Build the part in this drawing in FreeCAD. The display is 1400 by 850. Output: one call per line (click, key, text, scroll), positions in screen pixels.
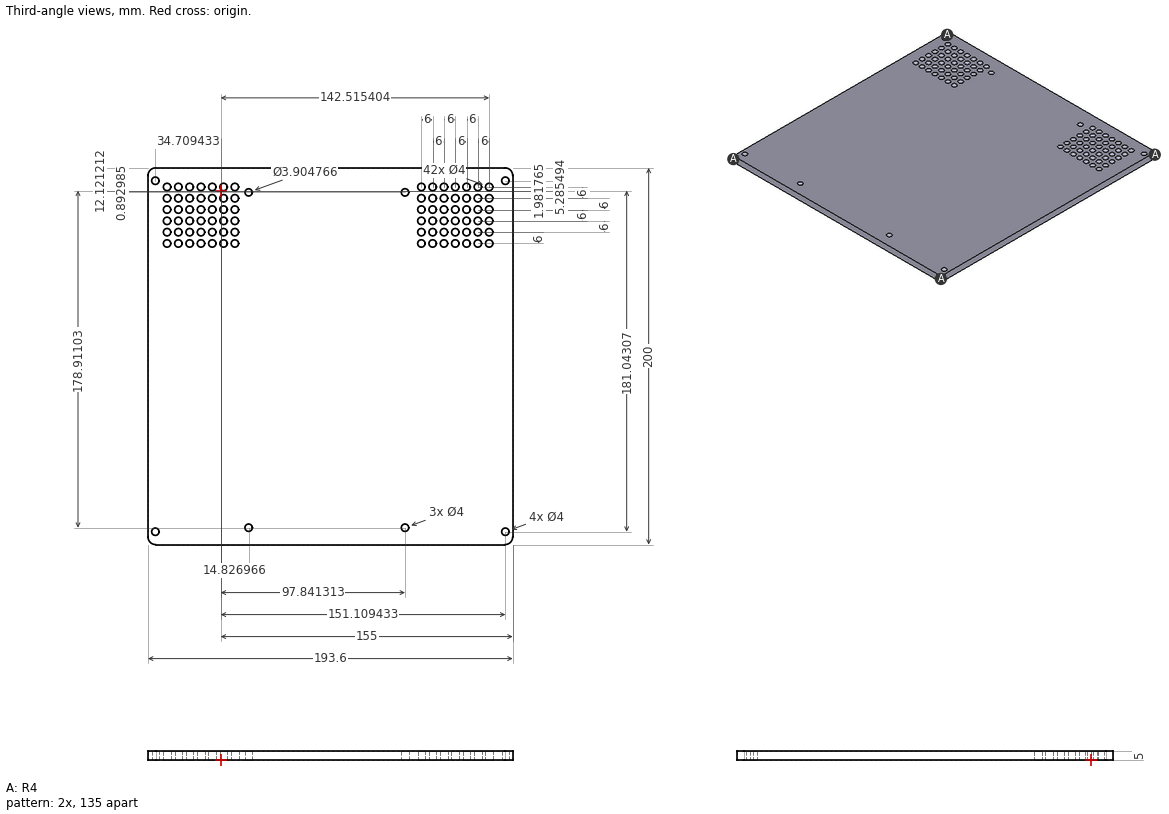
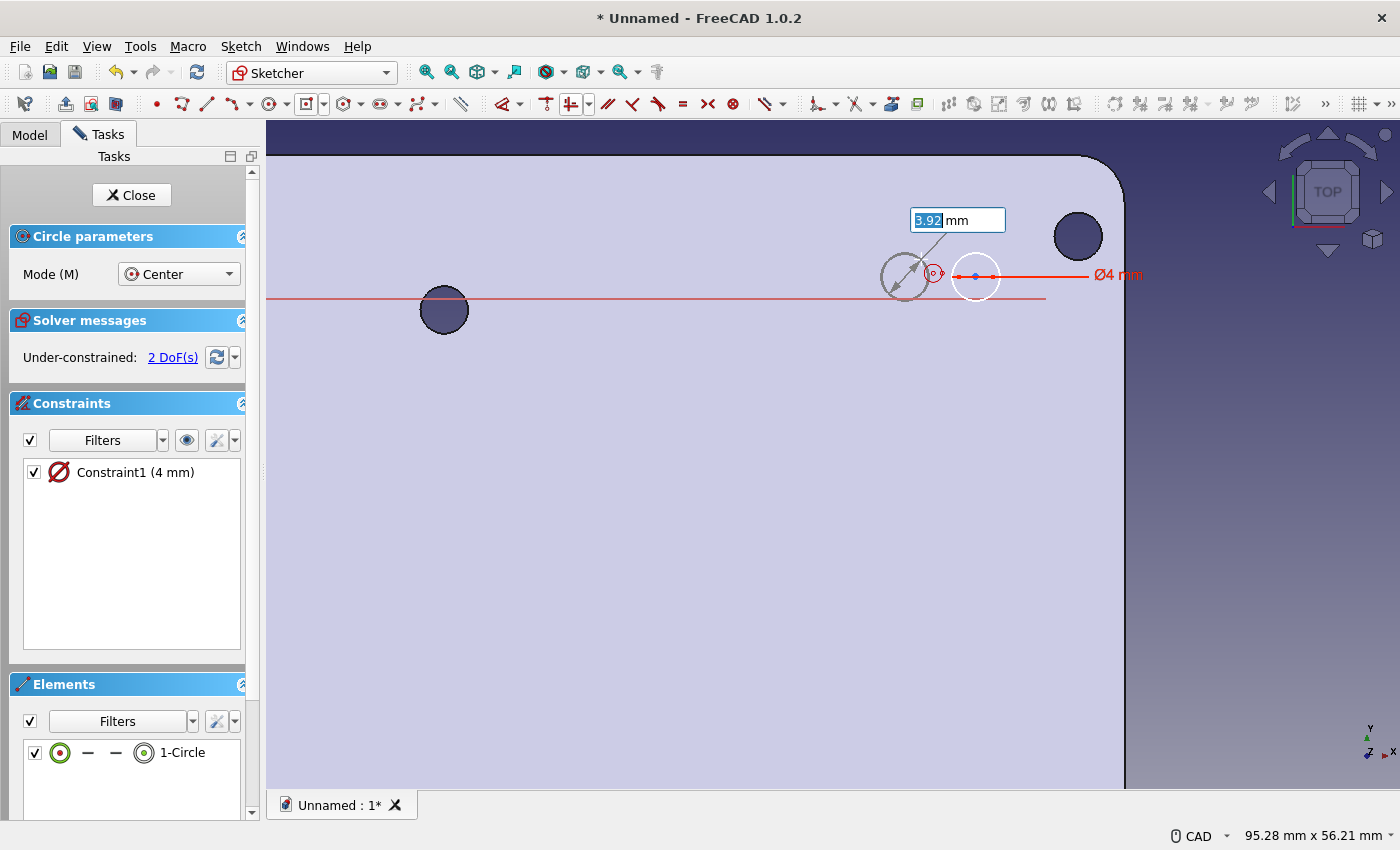
text(4)
key(Return)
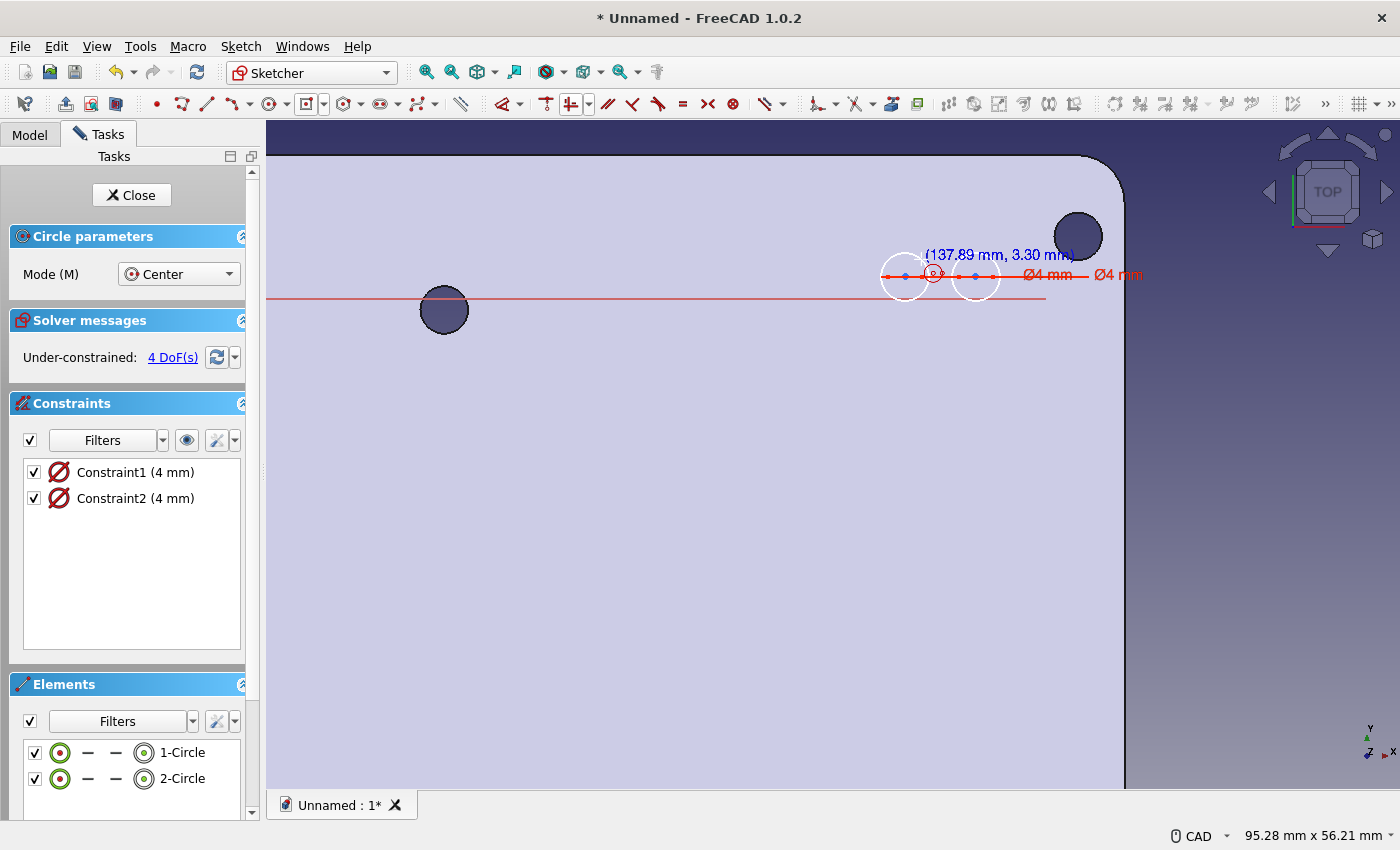
click(833, 276)
move(850, 259)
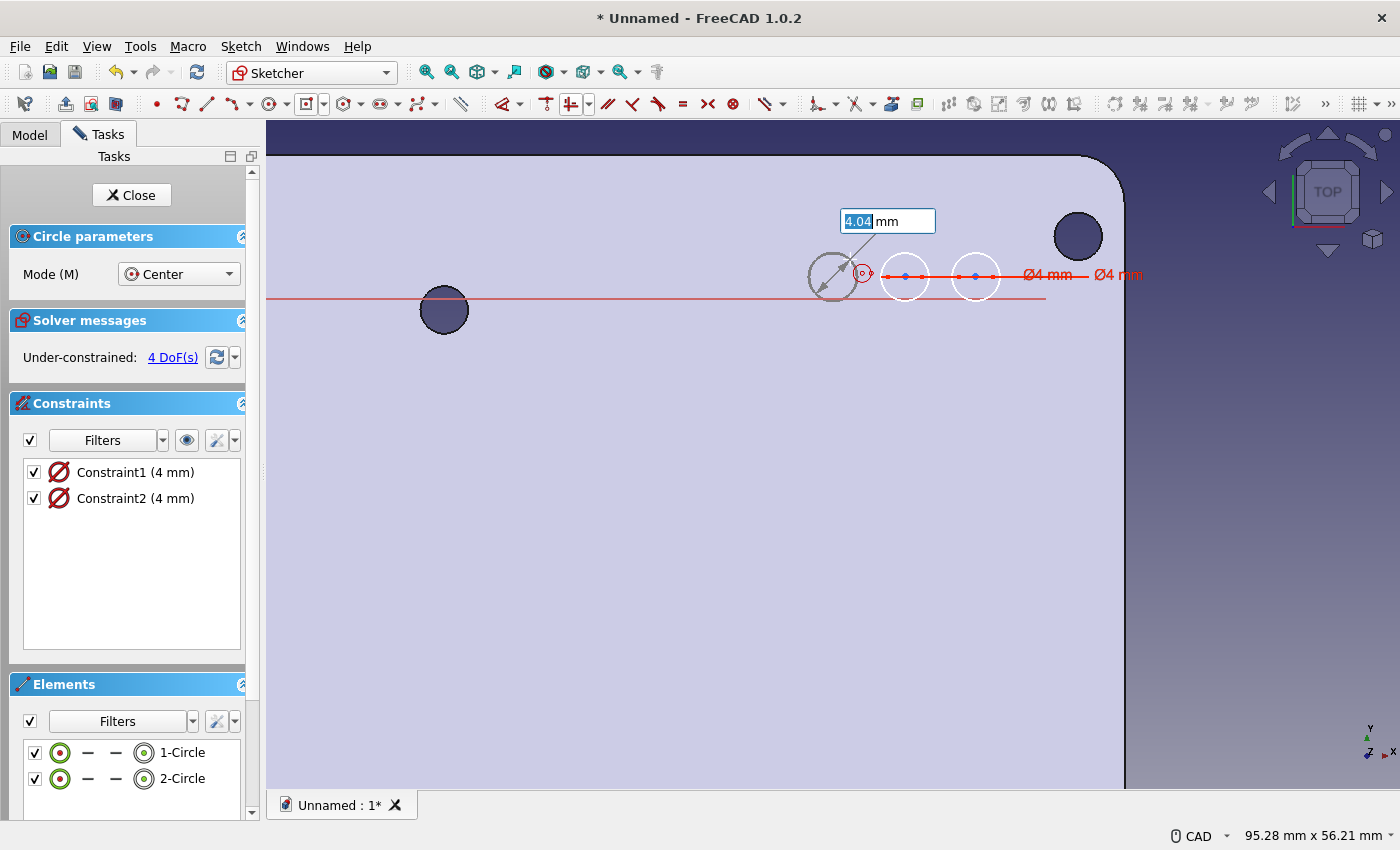
text(4)
key(Return)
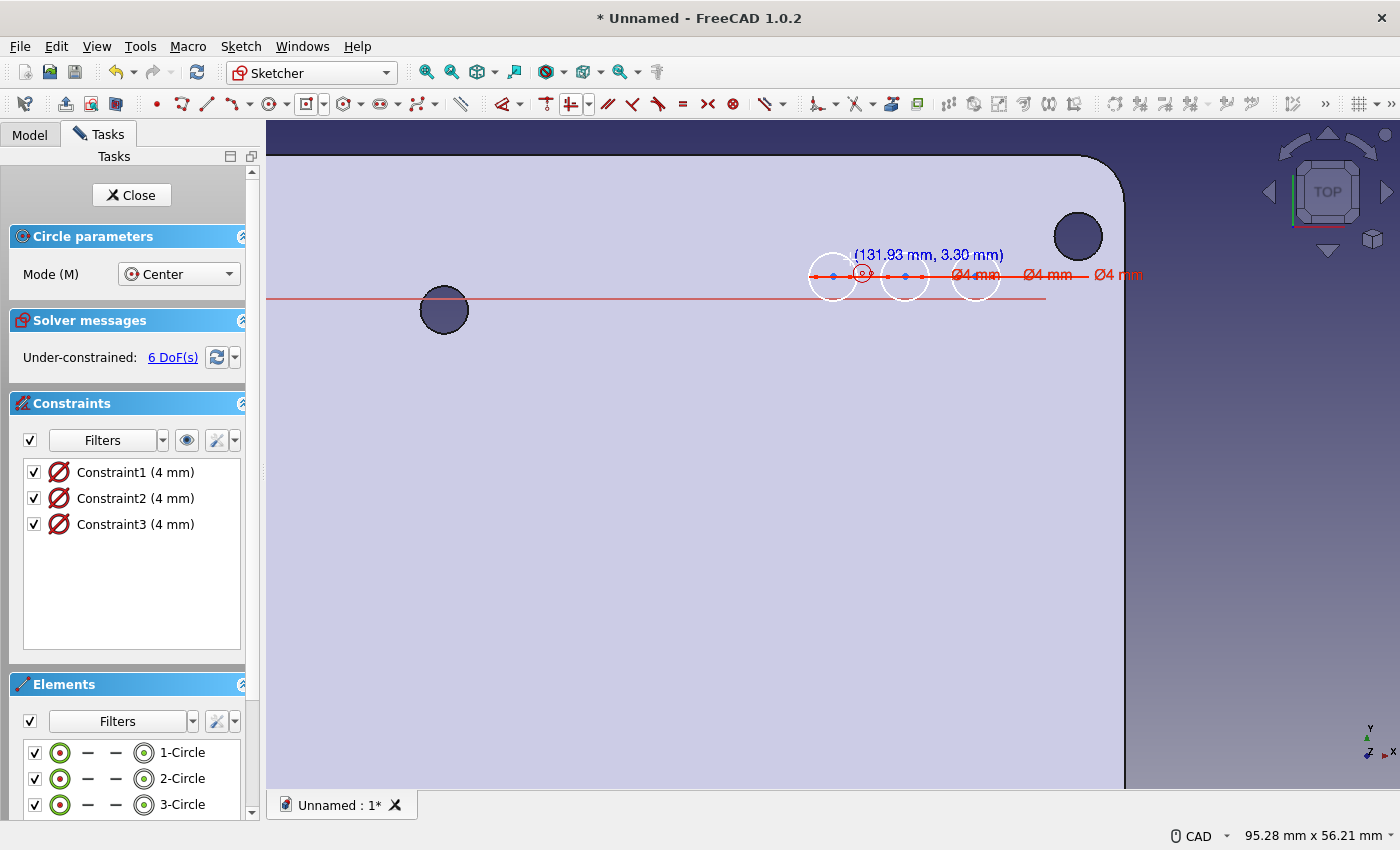
click(762, 276)
move(779, 259)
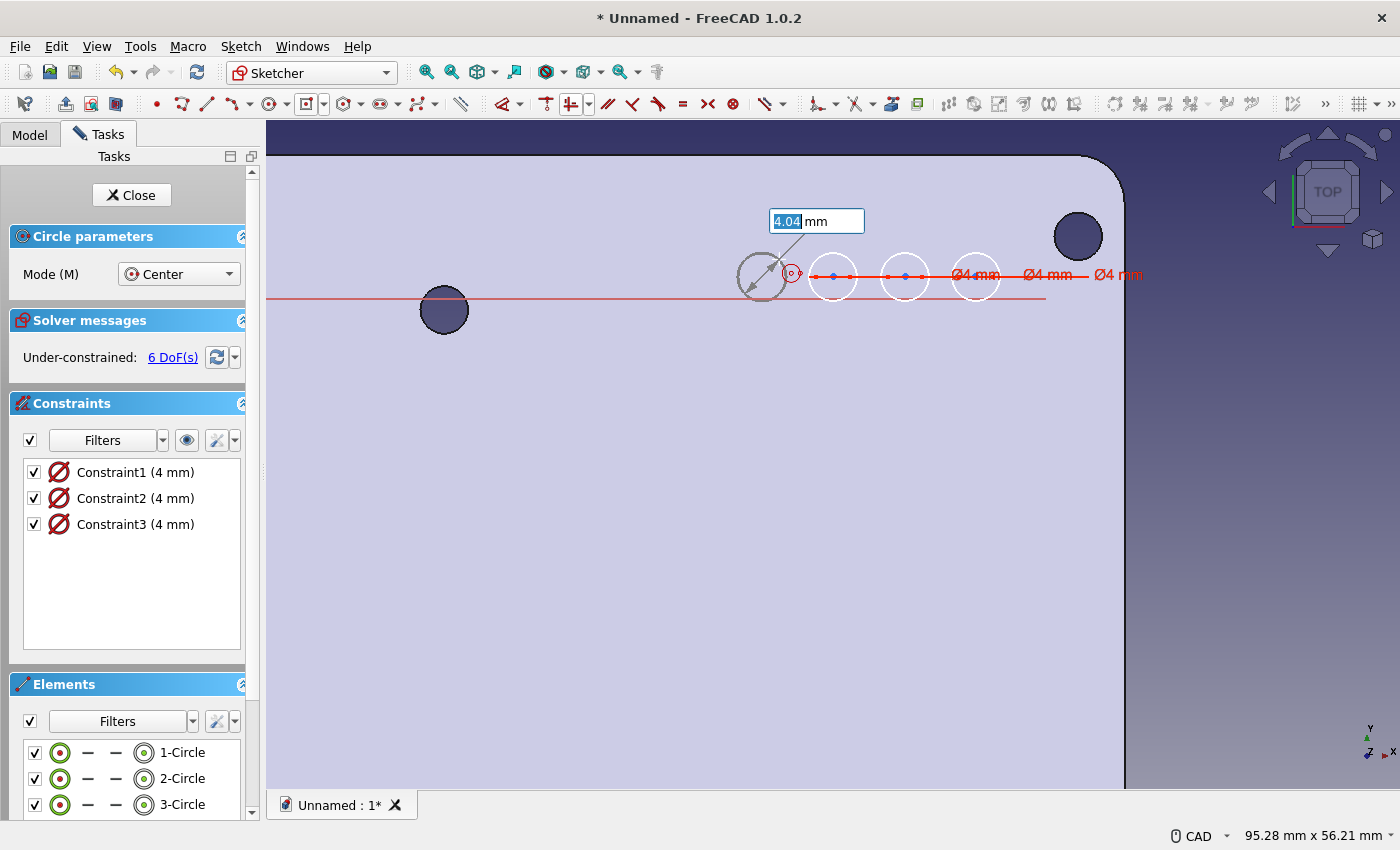
text(4)
key(Return)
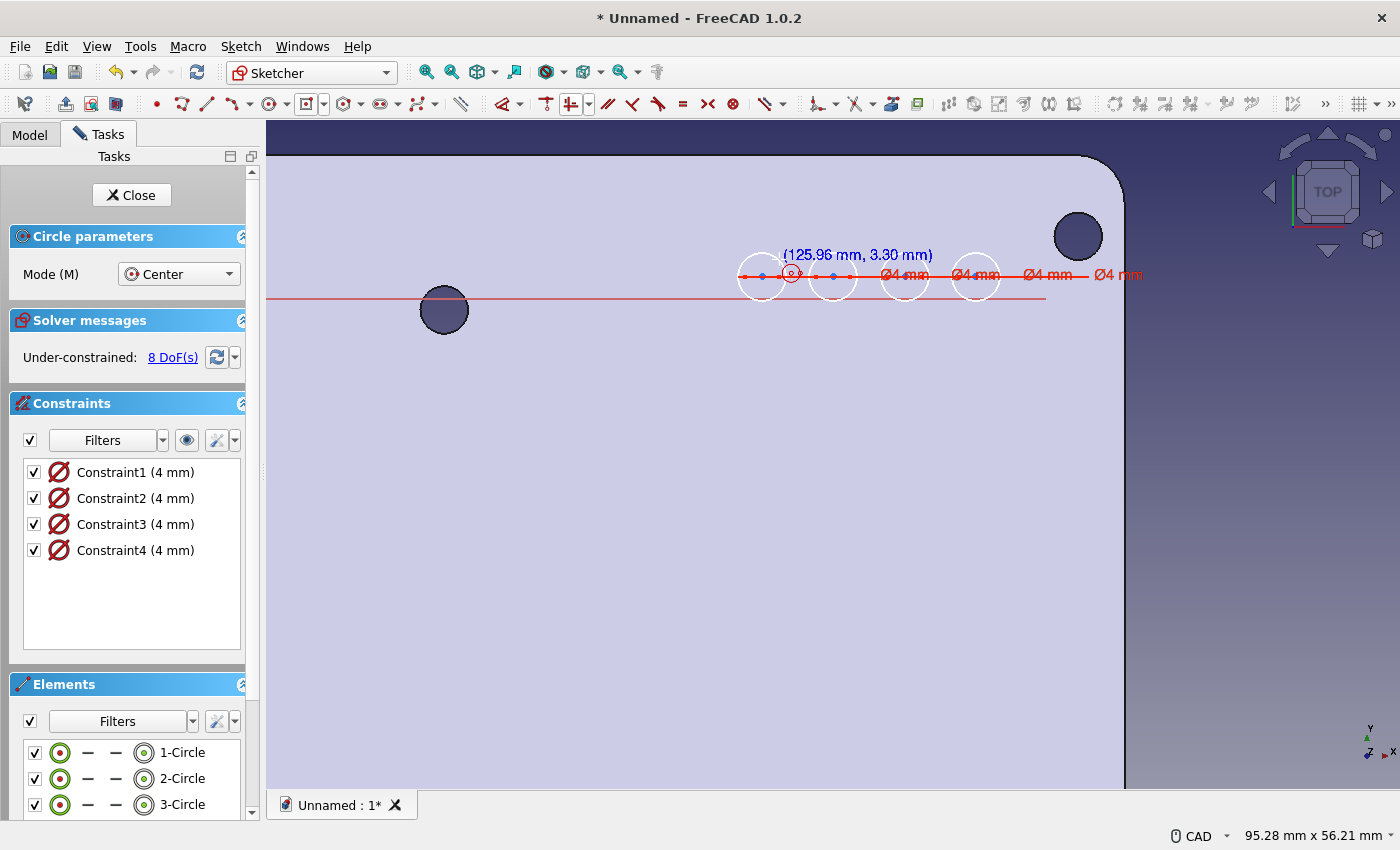
click(690, 276)
move(707, 259)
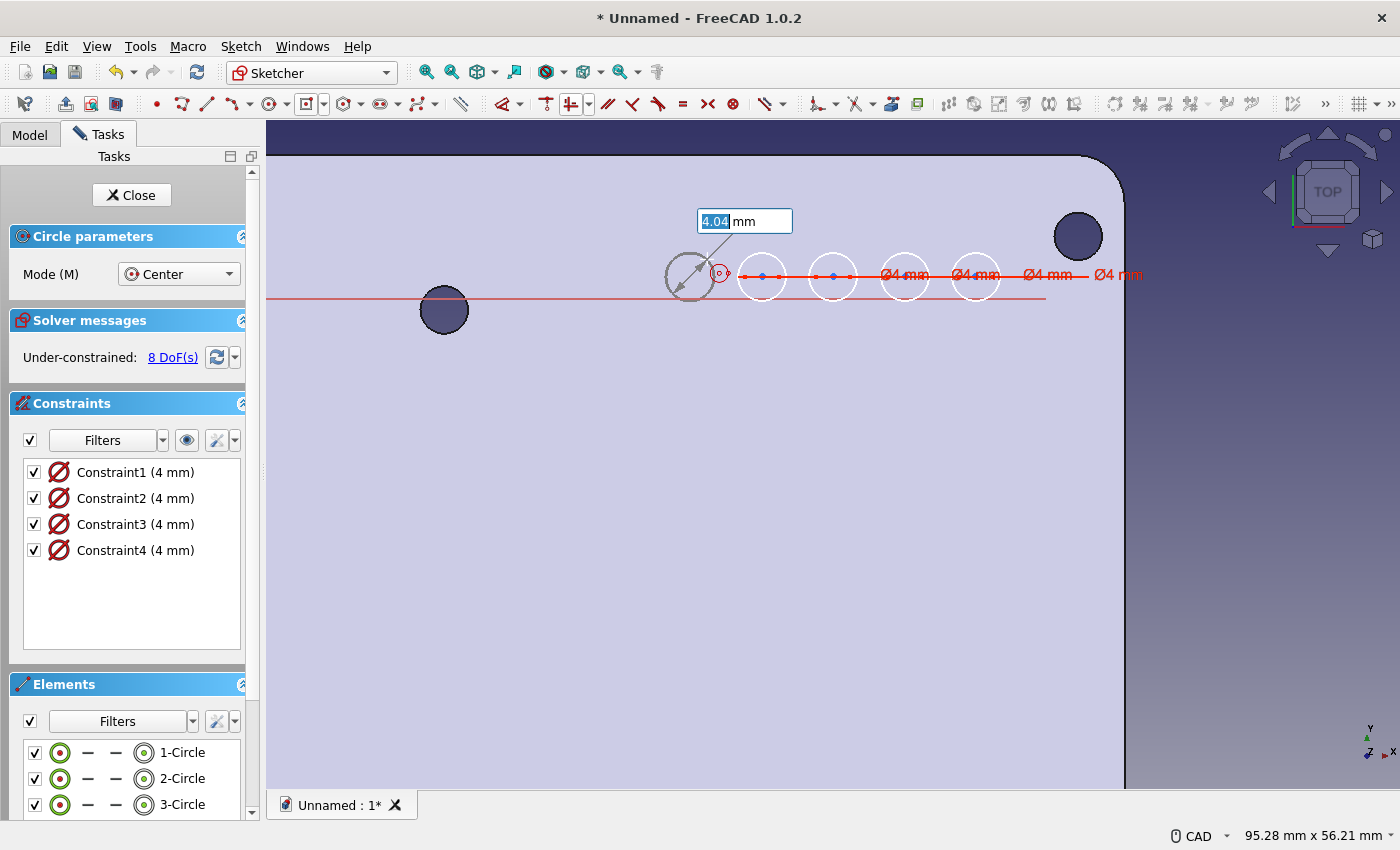
text(4)
key(Return)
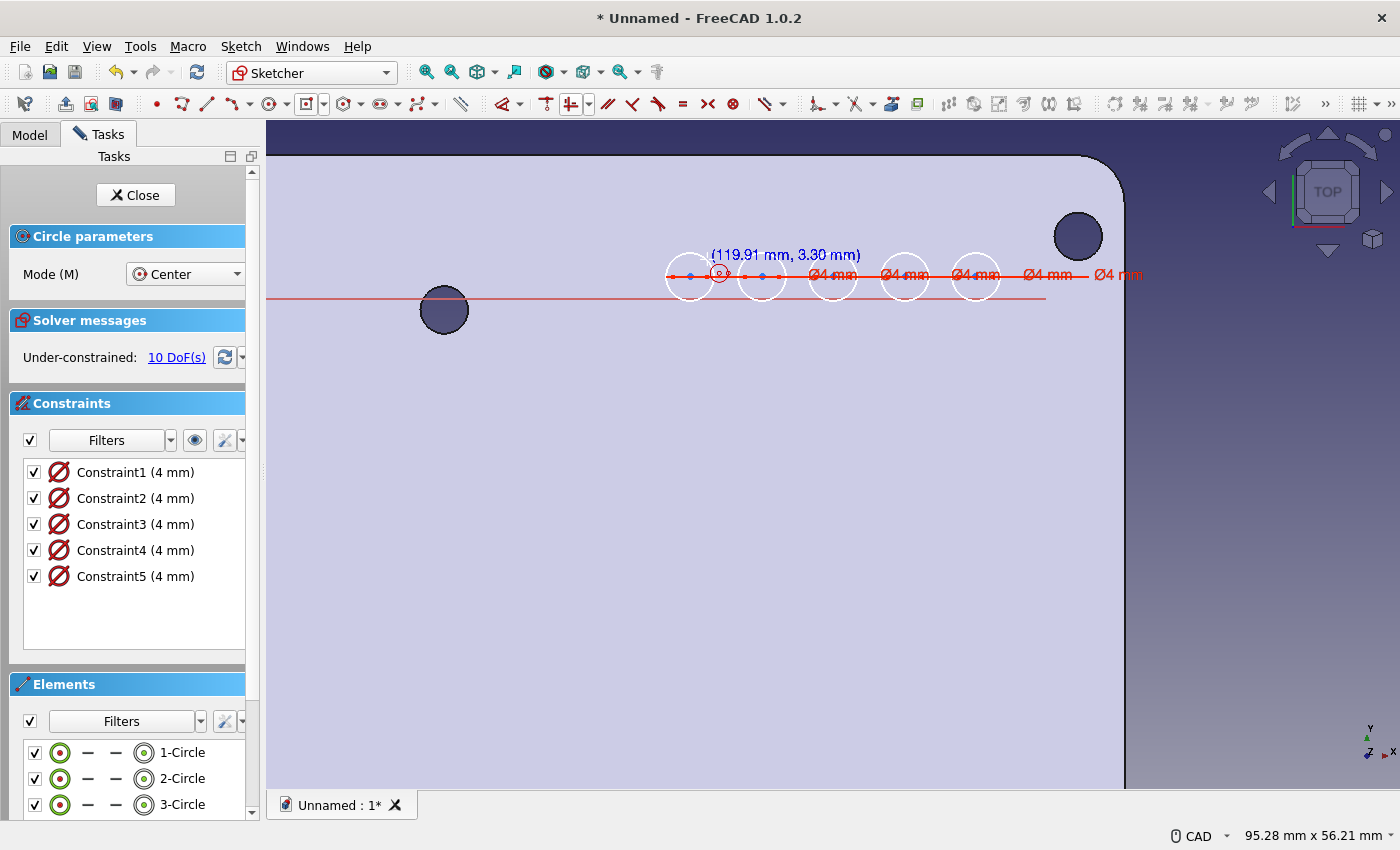
click(619, 276)
move(636, 259)